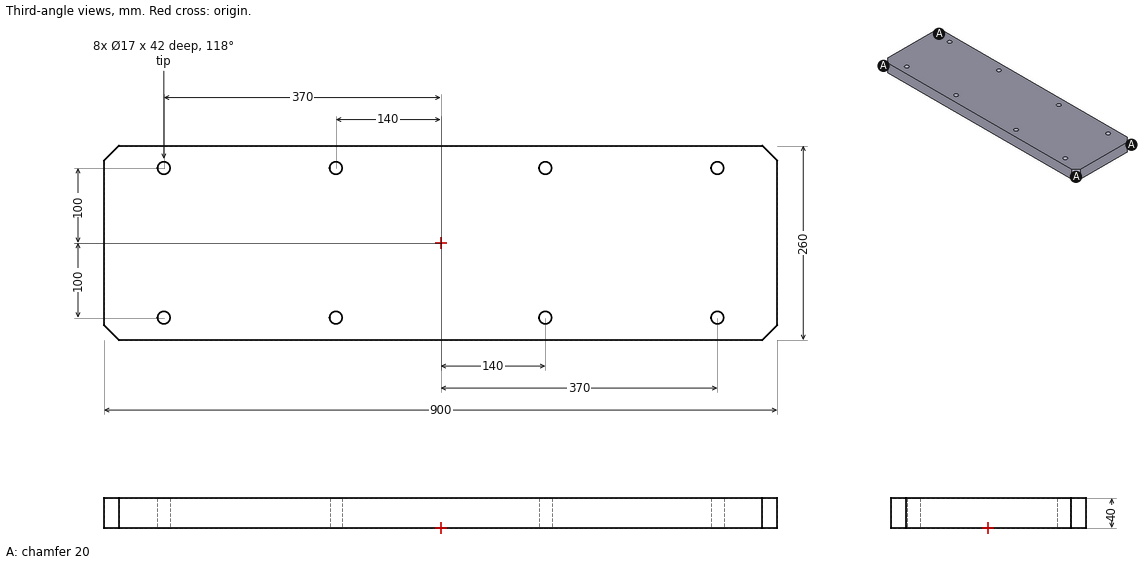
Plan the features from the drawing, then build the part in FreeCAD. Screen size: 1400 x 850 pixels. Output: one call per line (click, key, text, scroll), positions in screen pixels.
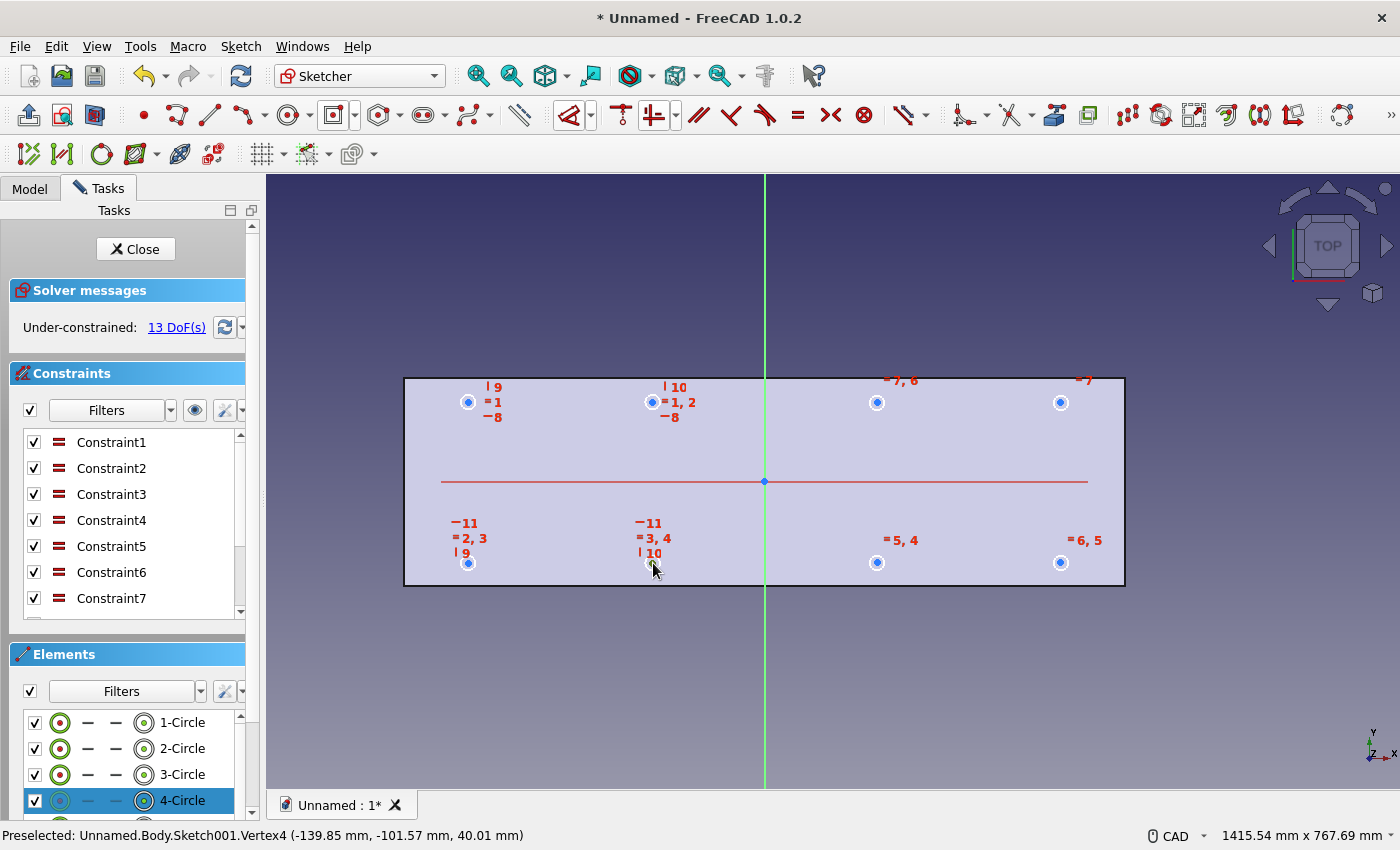
click(877, 563)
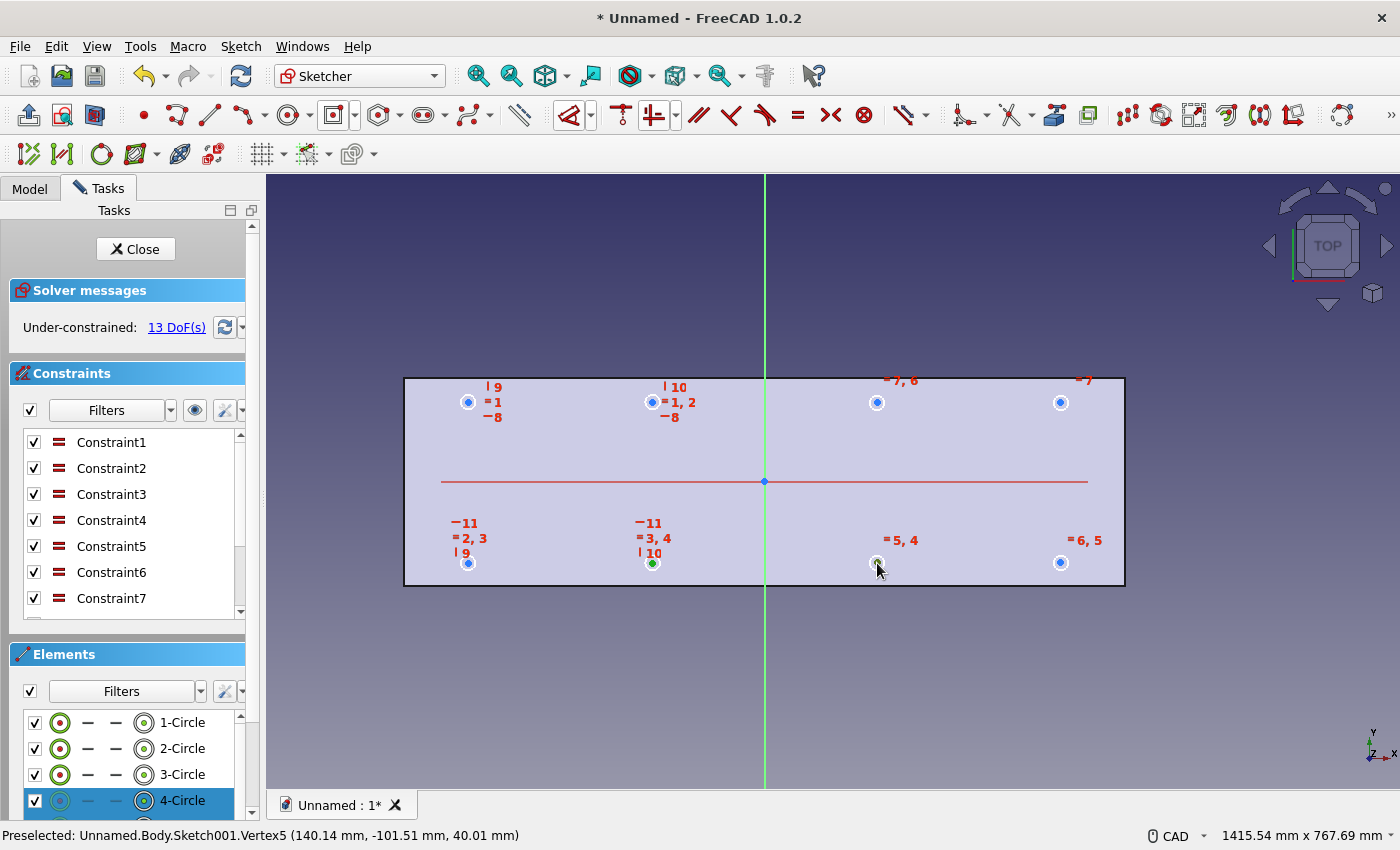
click(676, 116)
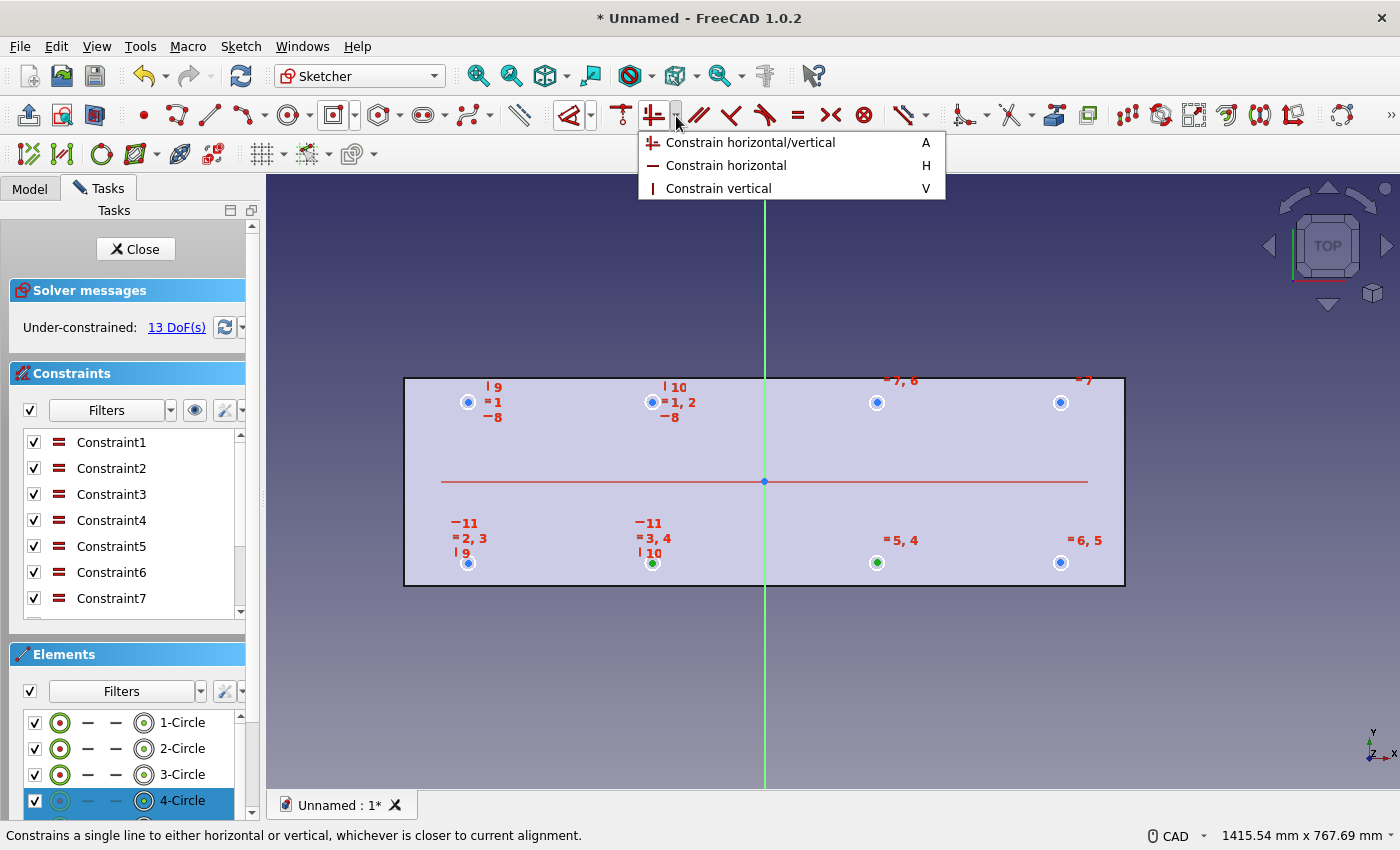
click(792, 166)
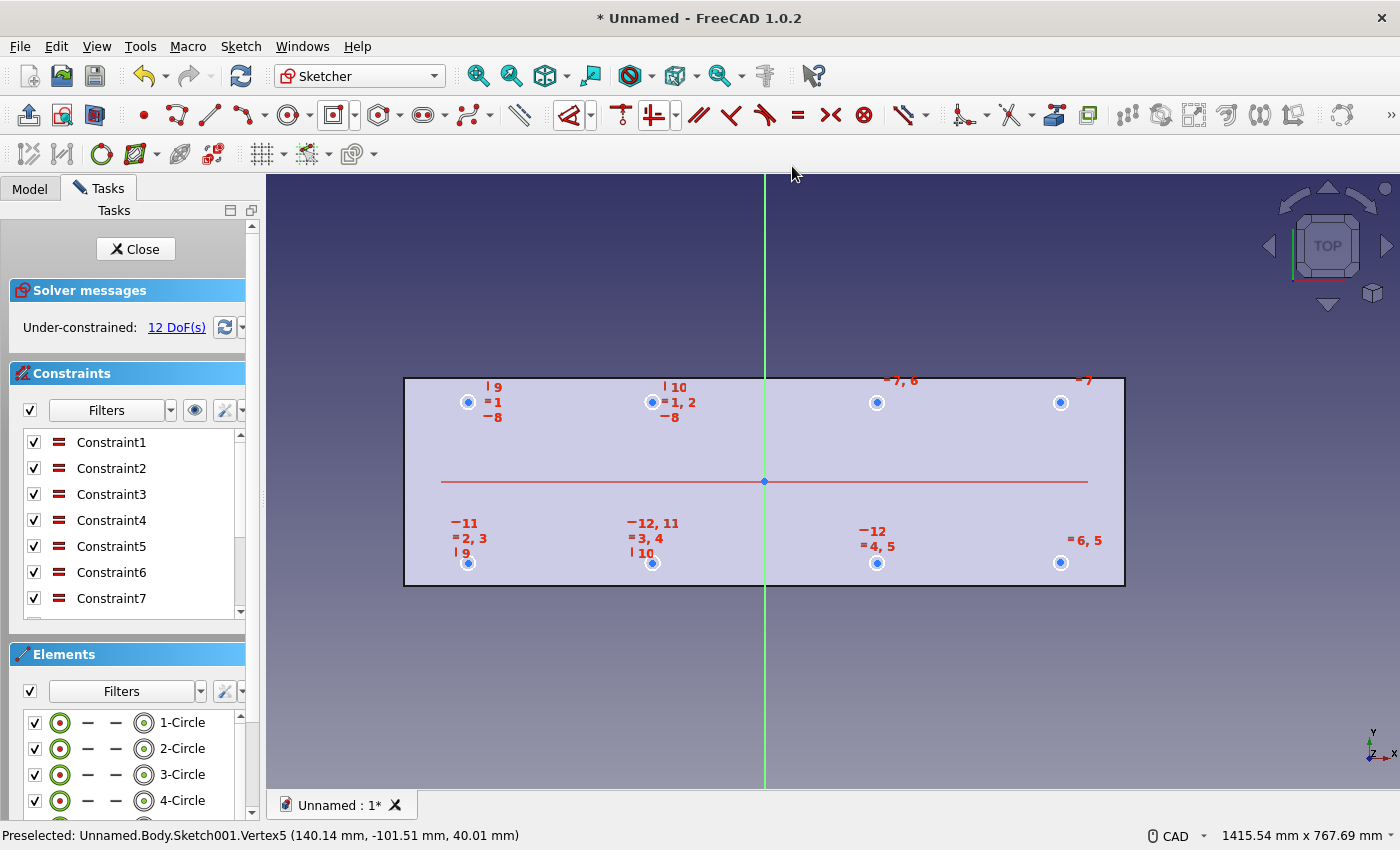
click(877, 563)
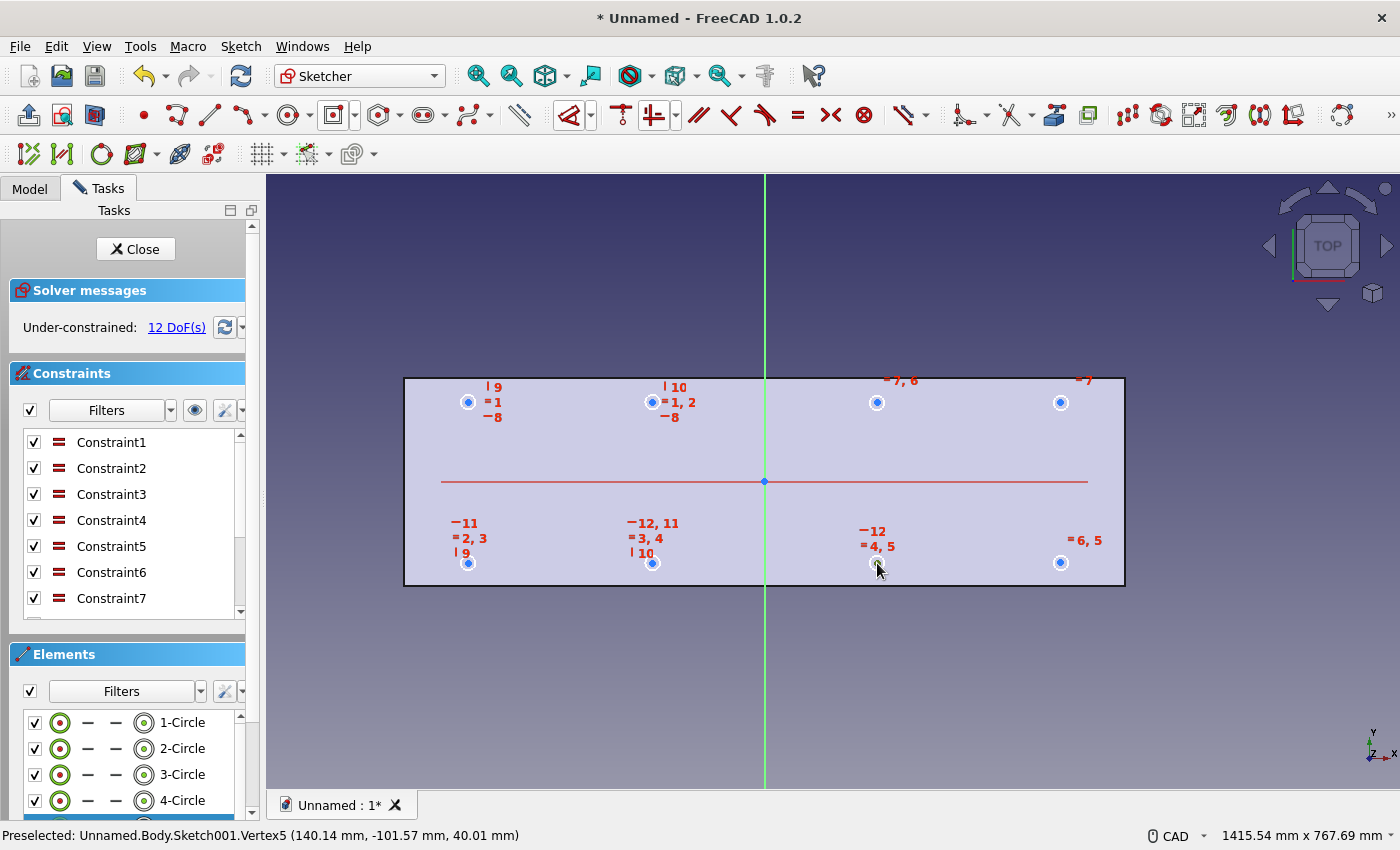
click(1061, 563)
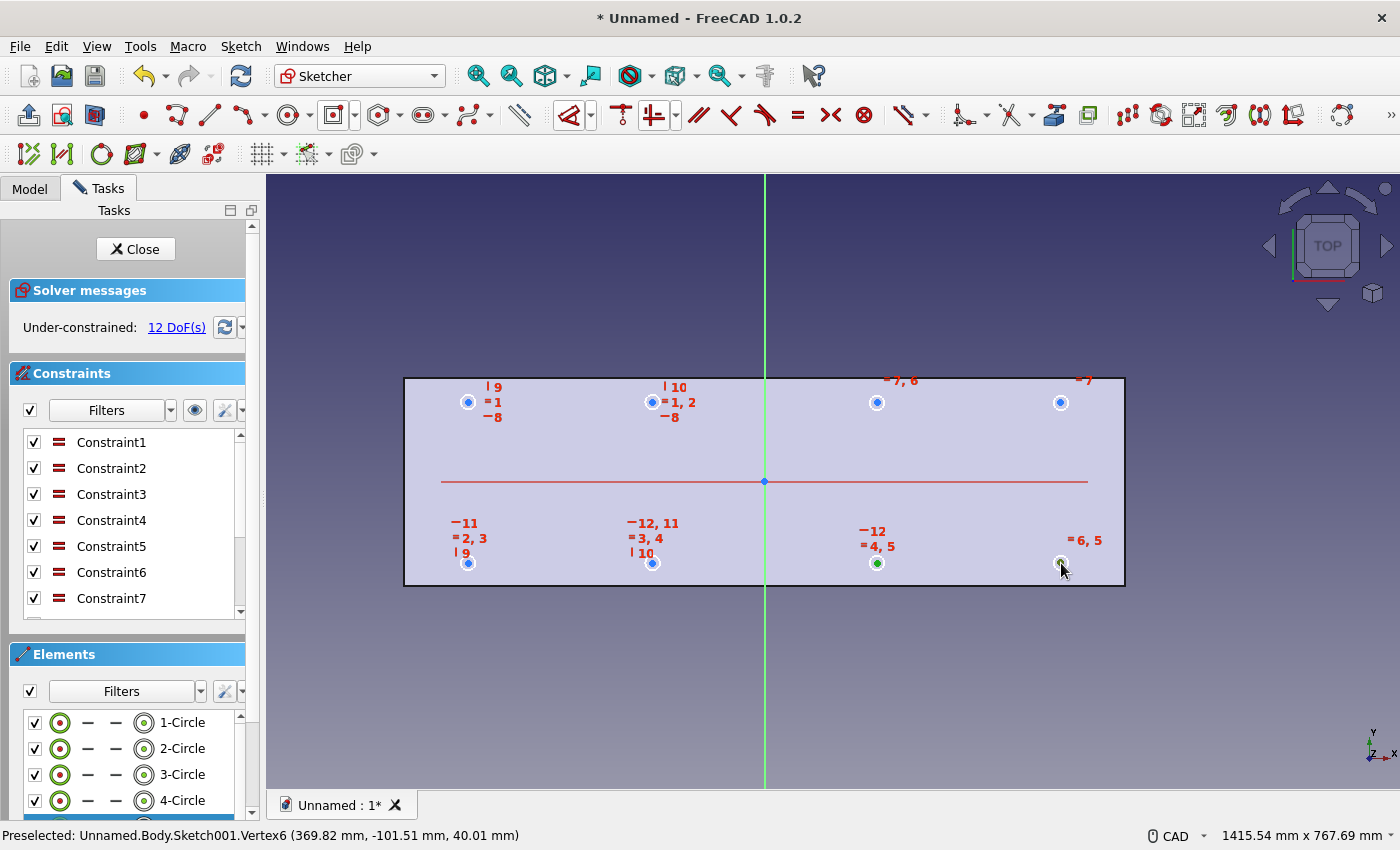
key(h)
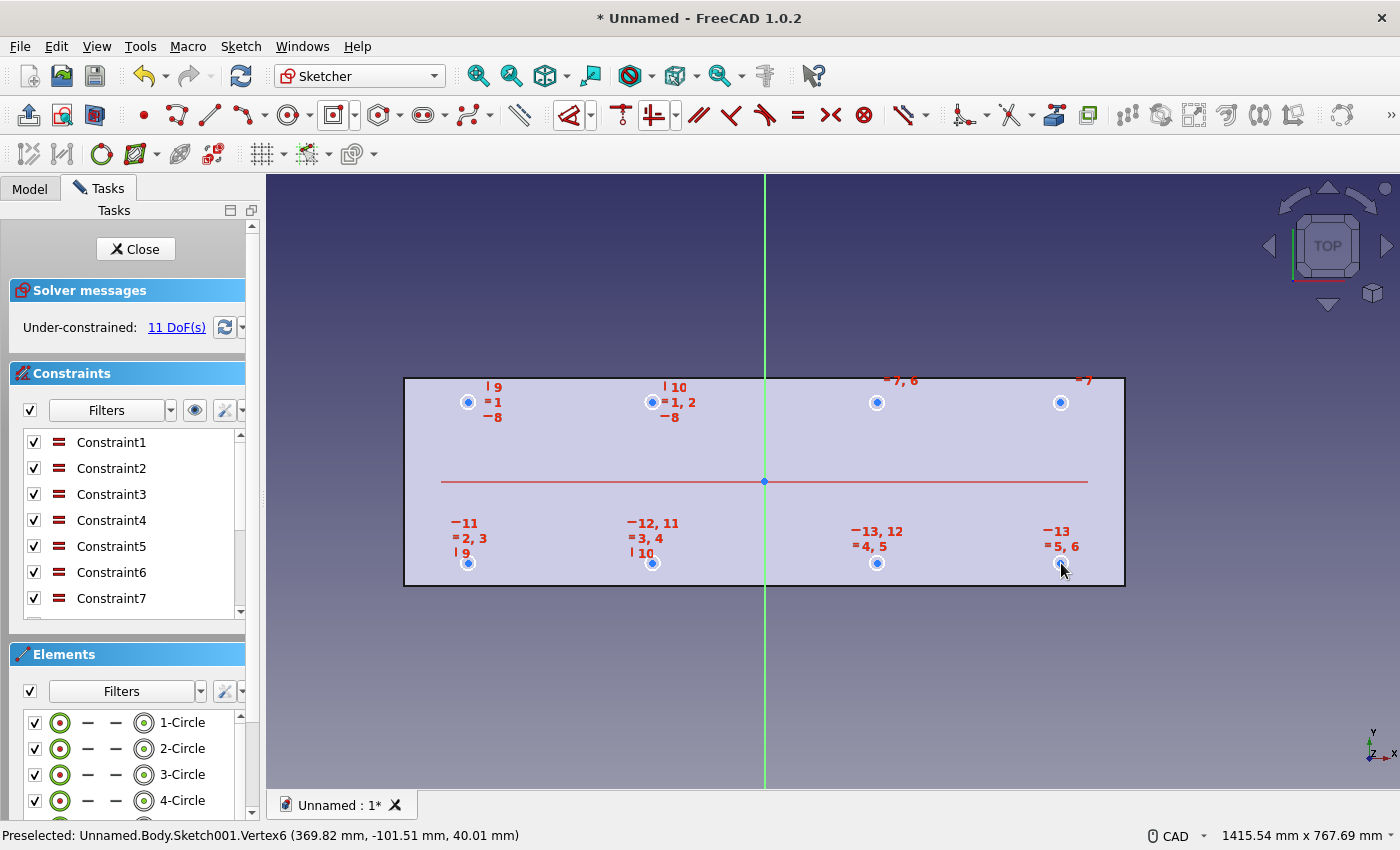
click(877, 563)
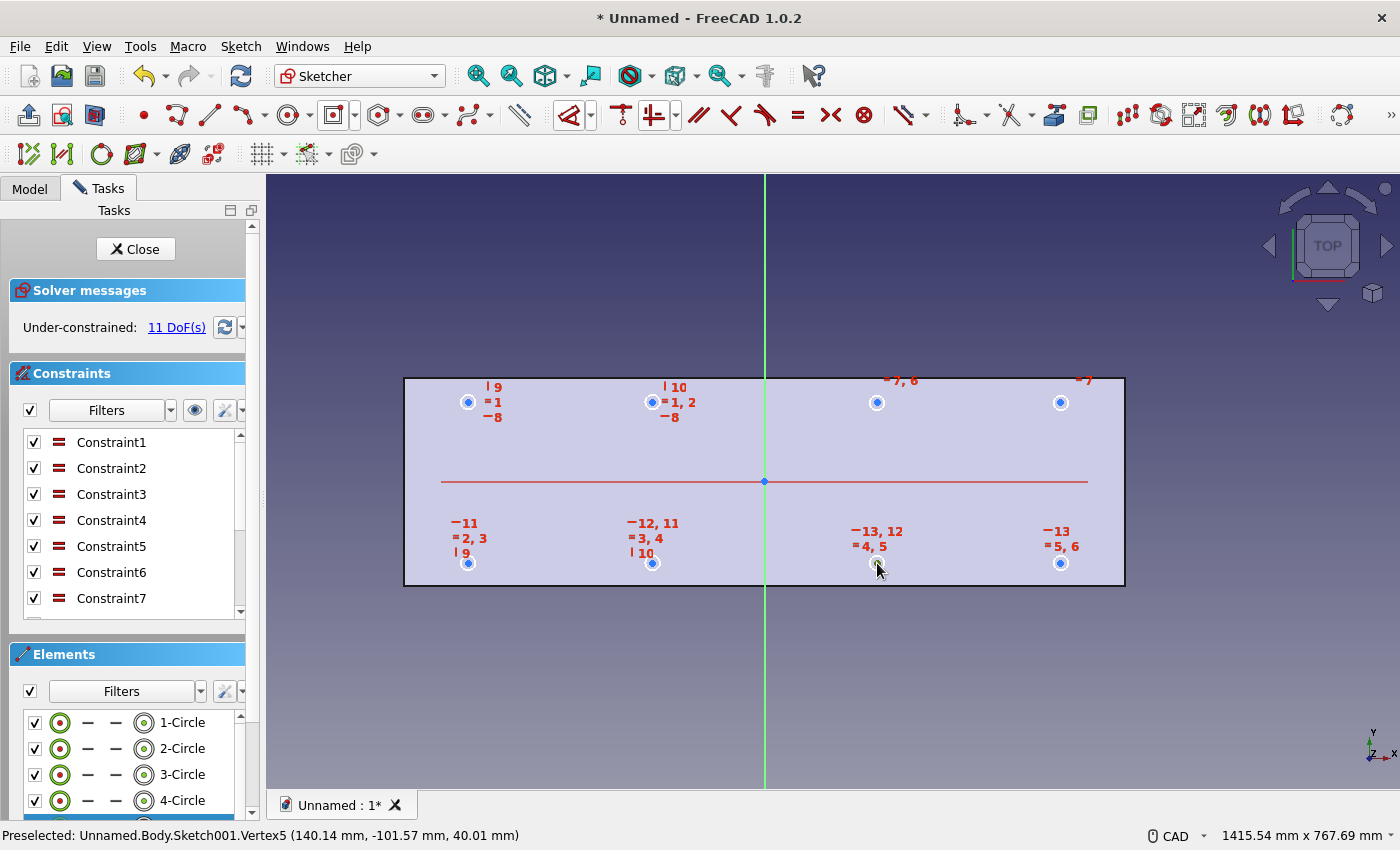
click(877, 403)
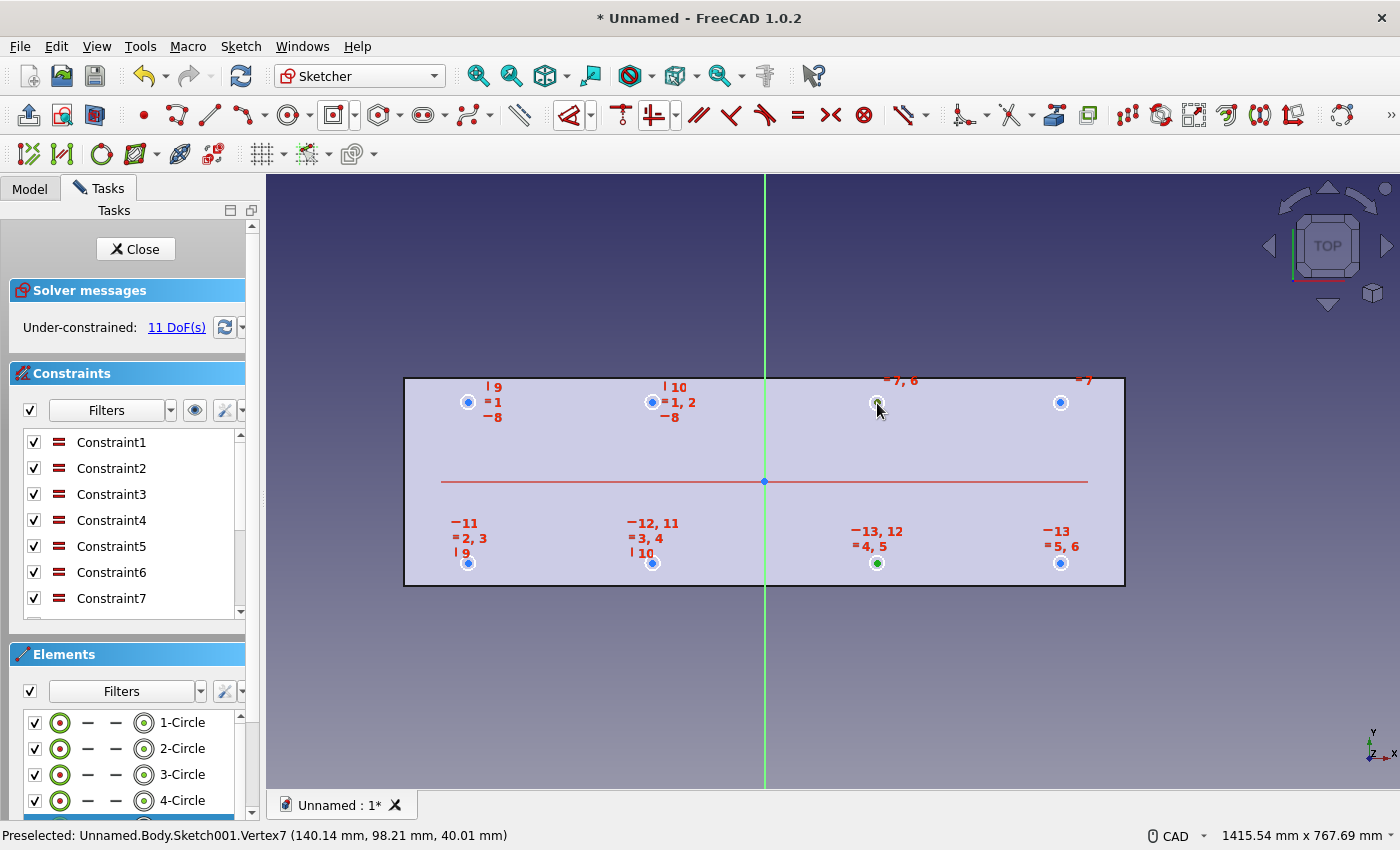
click(676, 116)